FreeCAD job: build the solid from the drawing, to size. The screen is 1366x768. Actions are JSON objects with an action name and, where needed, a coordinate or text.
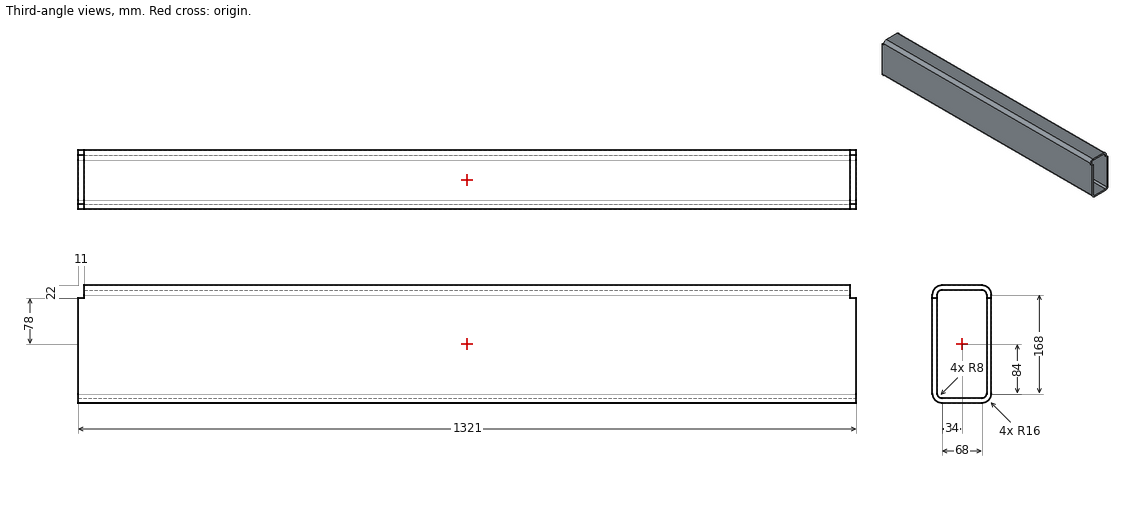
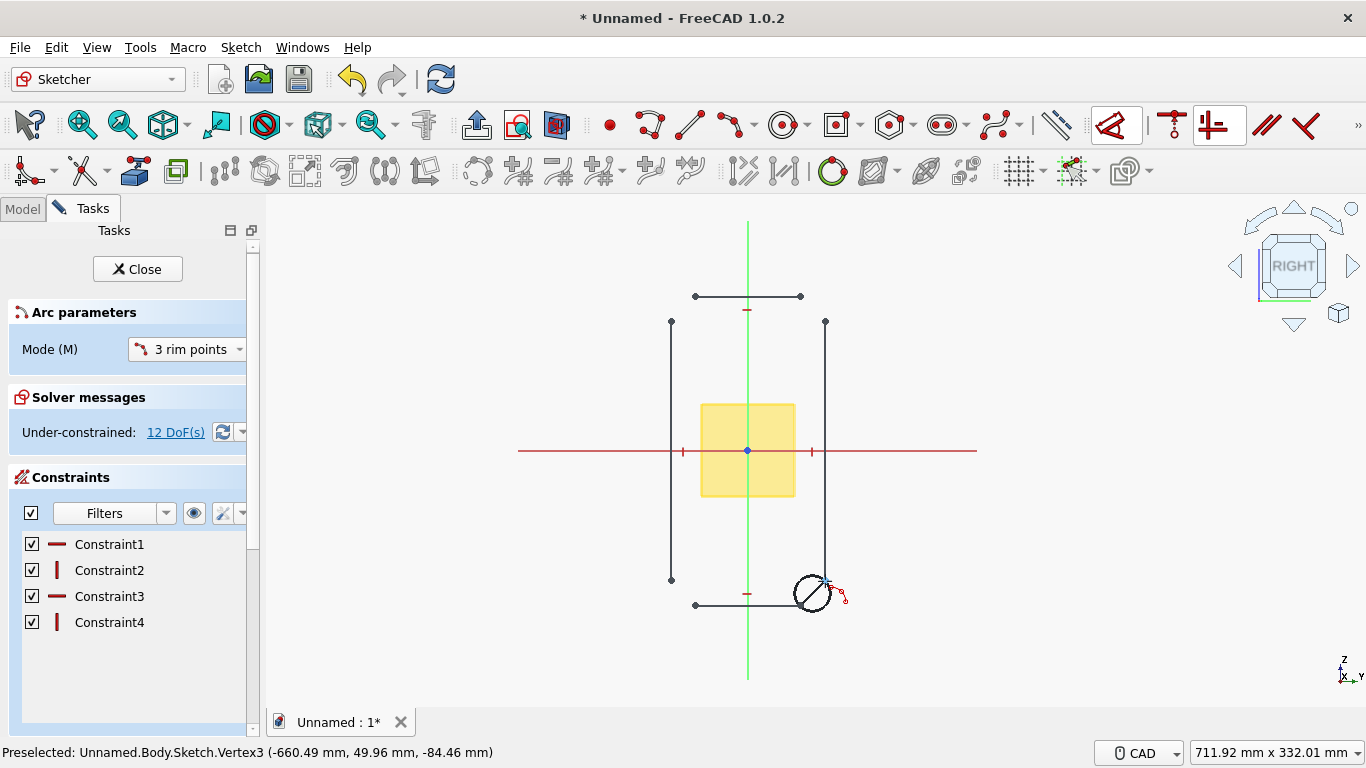
{"action": "scroll", "coordinate": [818, 598], "scroll_direction": "up", "scroll_amount": 4}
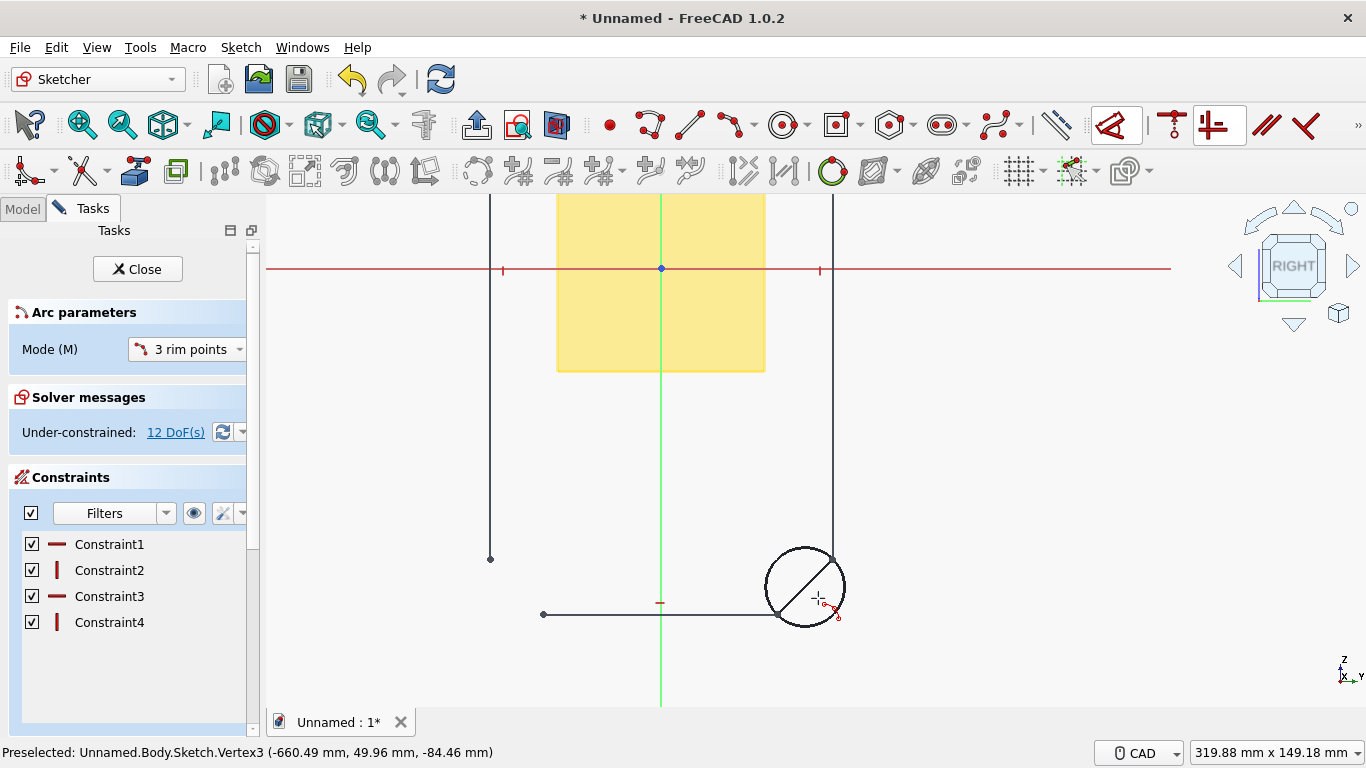
{"action": "left_click", "coordinate": [817, 597]}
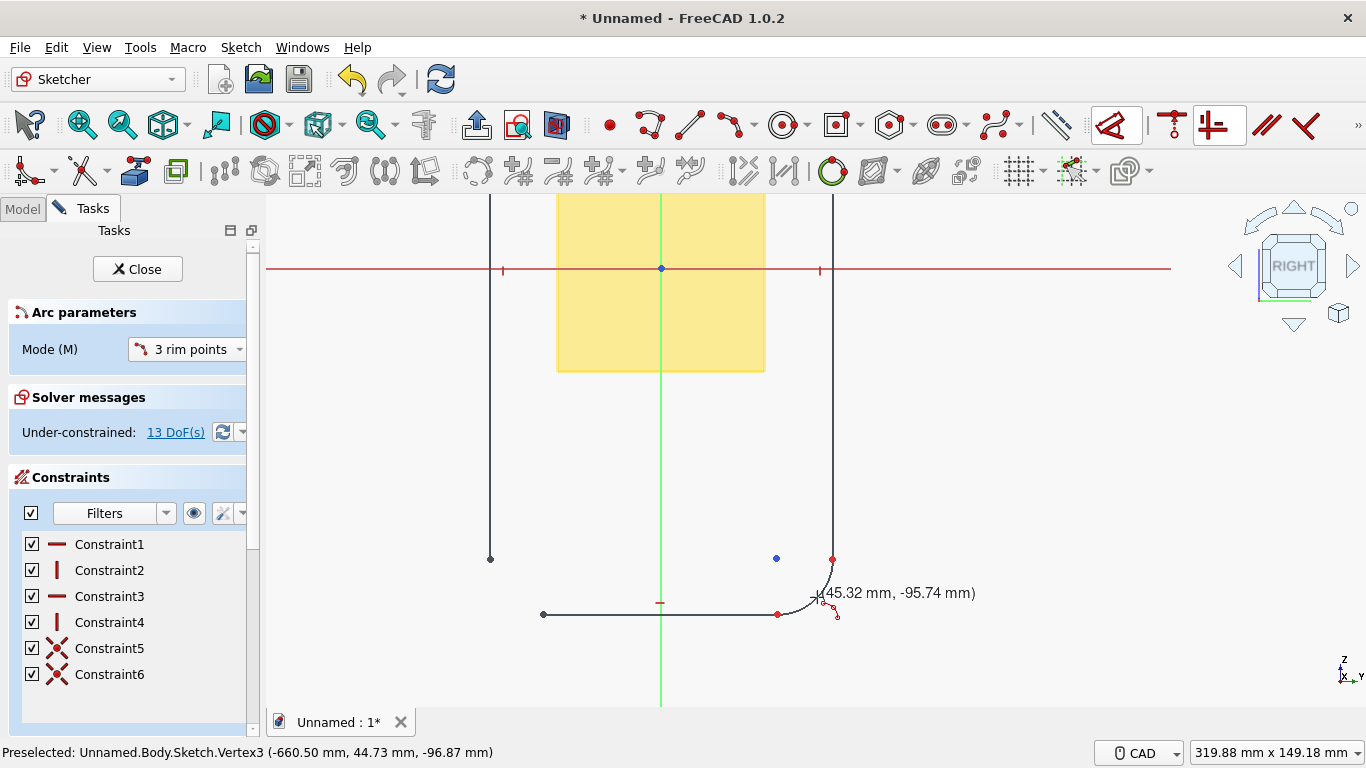
{"action": "scroll", "coordinate": [818, 599], "scroll_direction": "down", "scroll_amount": 4}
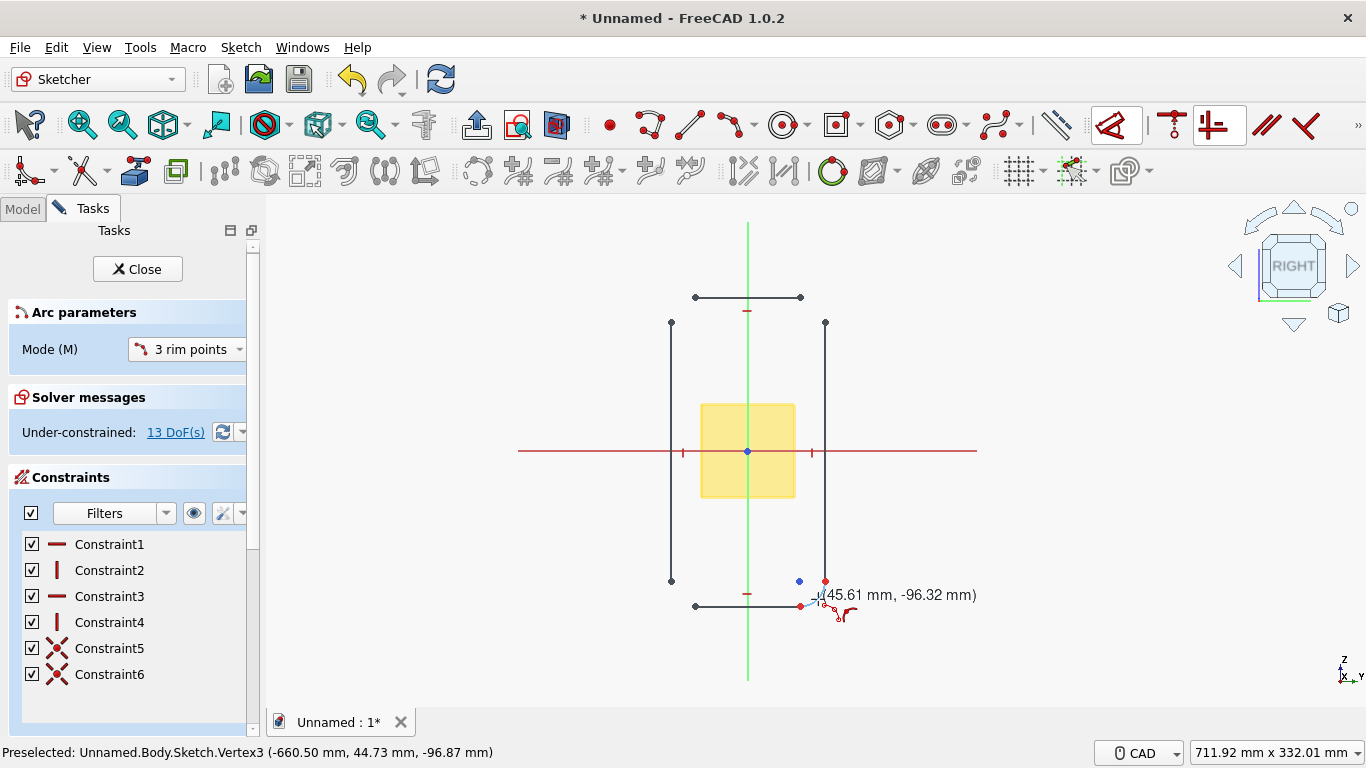
{"action": "left_click", "coordinate": [825, 323]}
{"action": "left_click", "coordinate": [800, 298]}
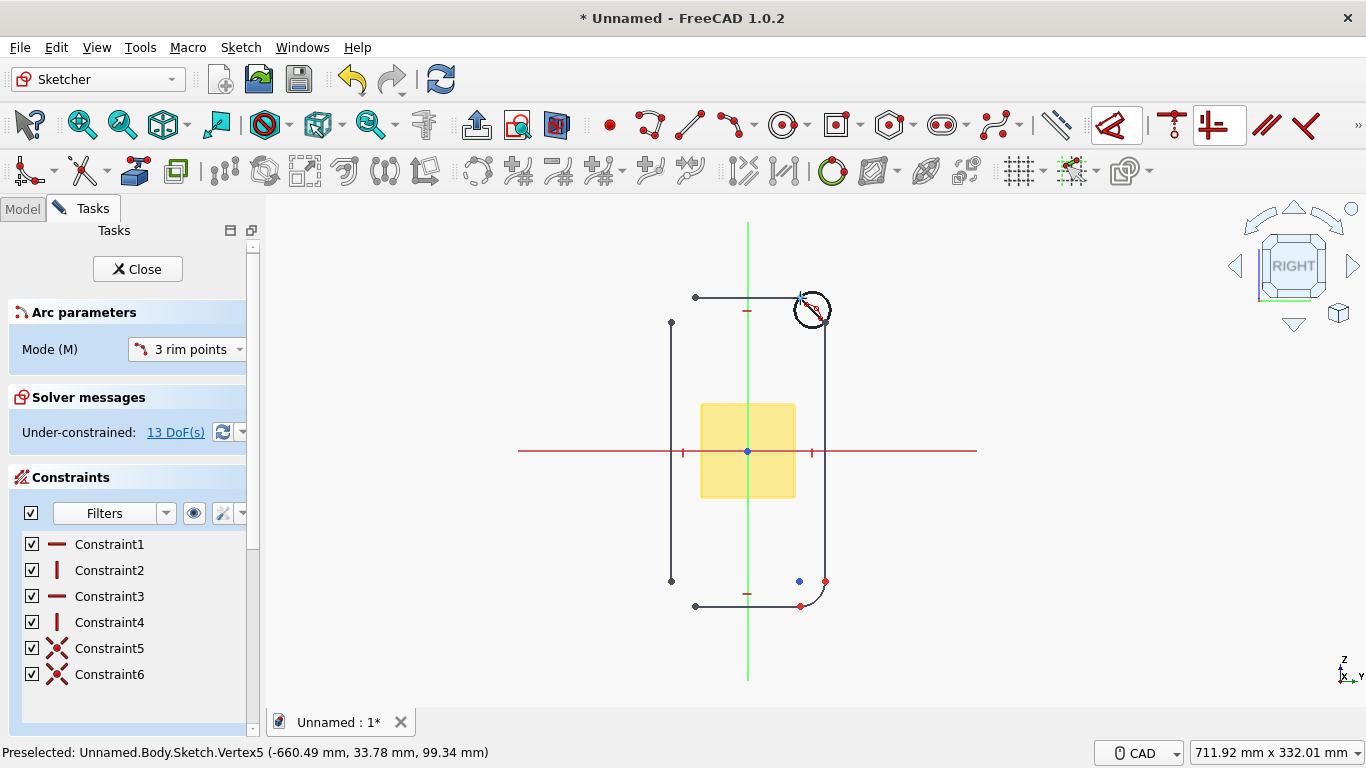
{"action": "scroll", "coordinate": [818, 304], "scroll_direction": "up", "scroll_amount": 4}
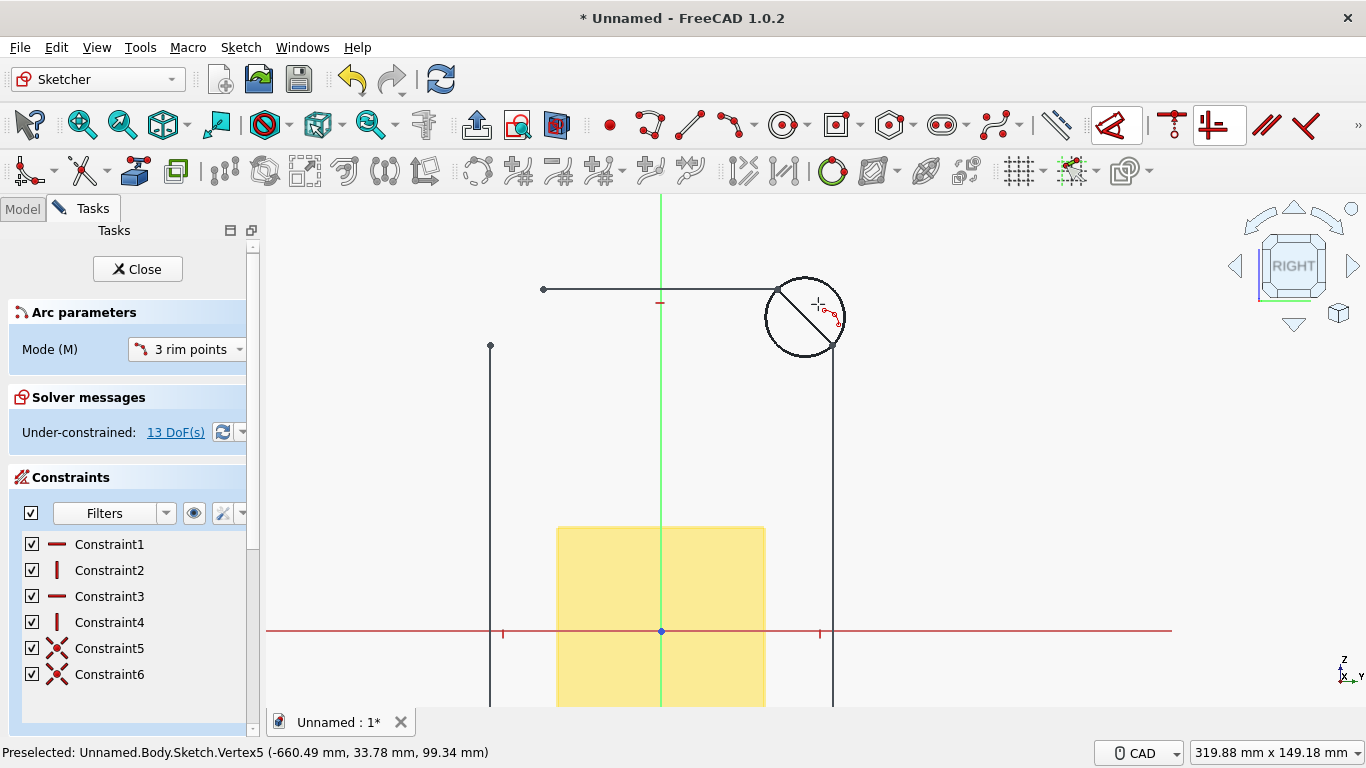
{"action": "left_click", "coordinate": [817, 303]}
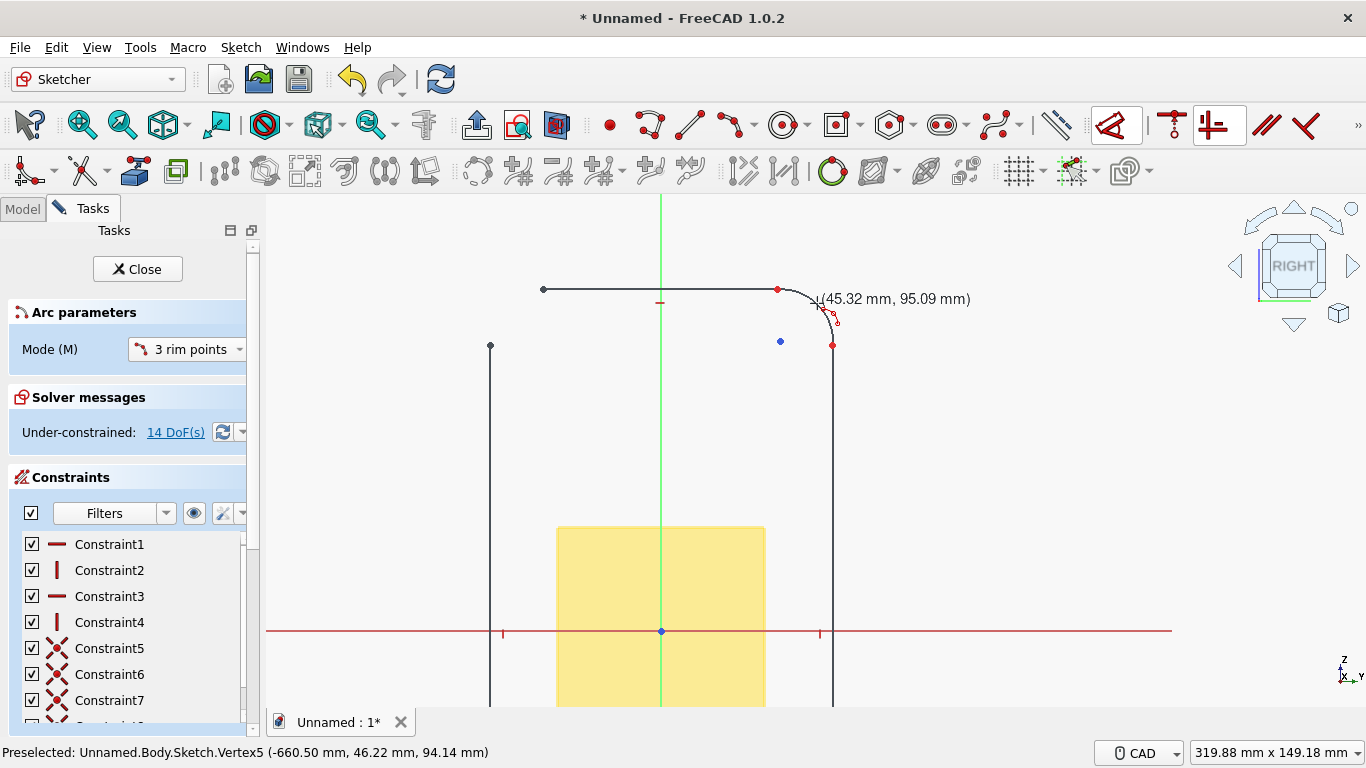
{"action": "left_click", "coordinate": [544, 289]}
{"action": "left_click", "coordinate": [490, 345]}
{"action": "left_click", "coordinate": [505, 303]}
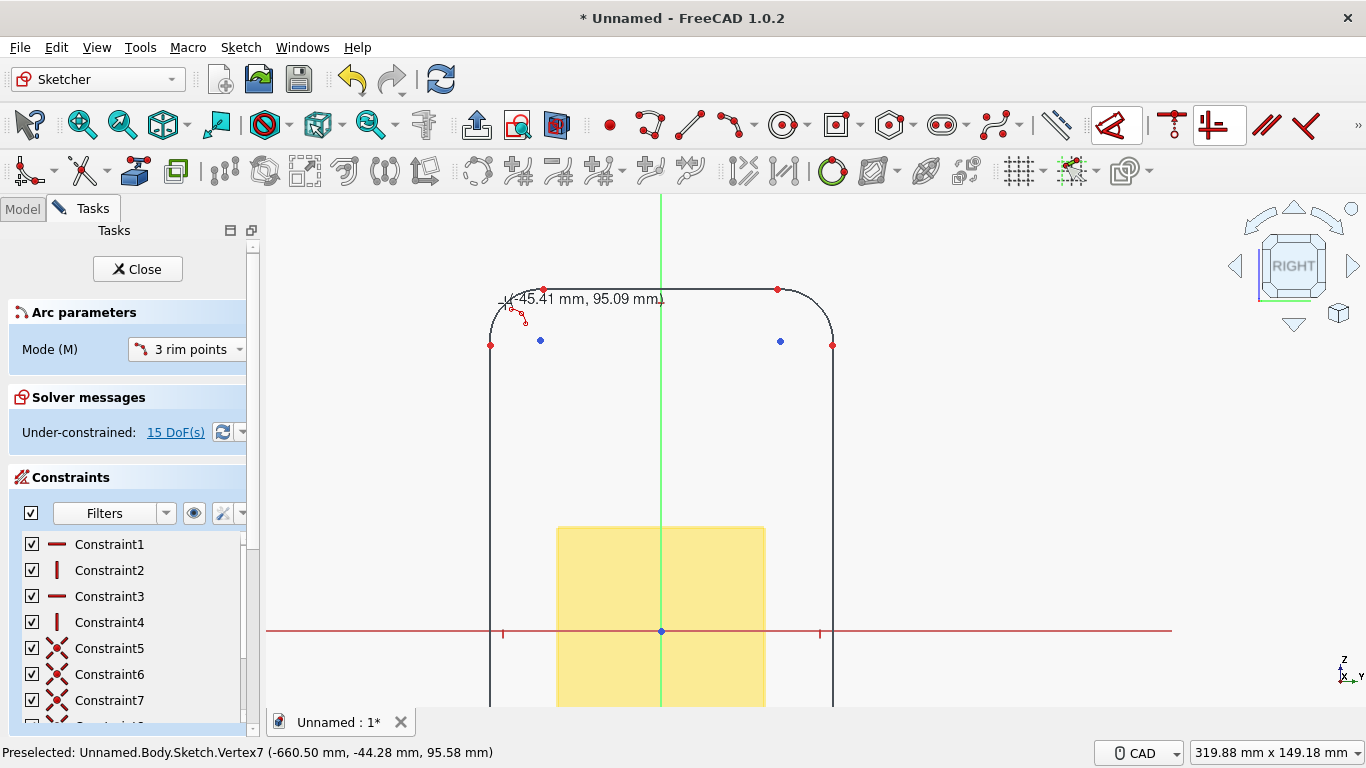
{"action": "scroll", "coordinate": [818, 303], "scroll_direction": "down", "scroll_amount": 4}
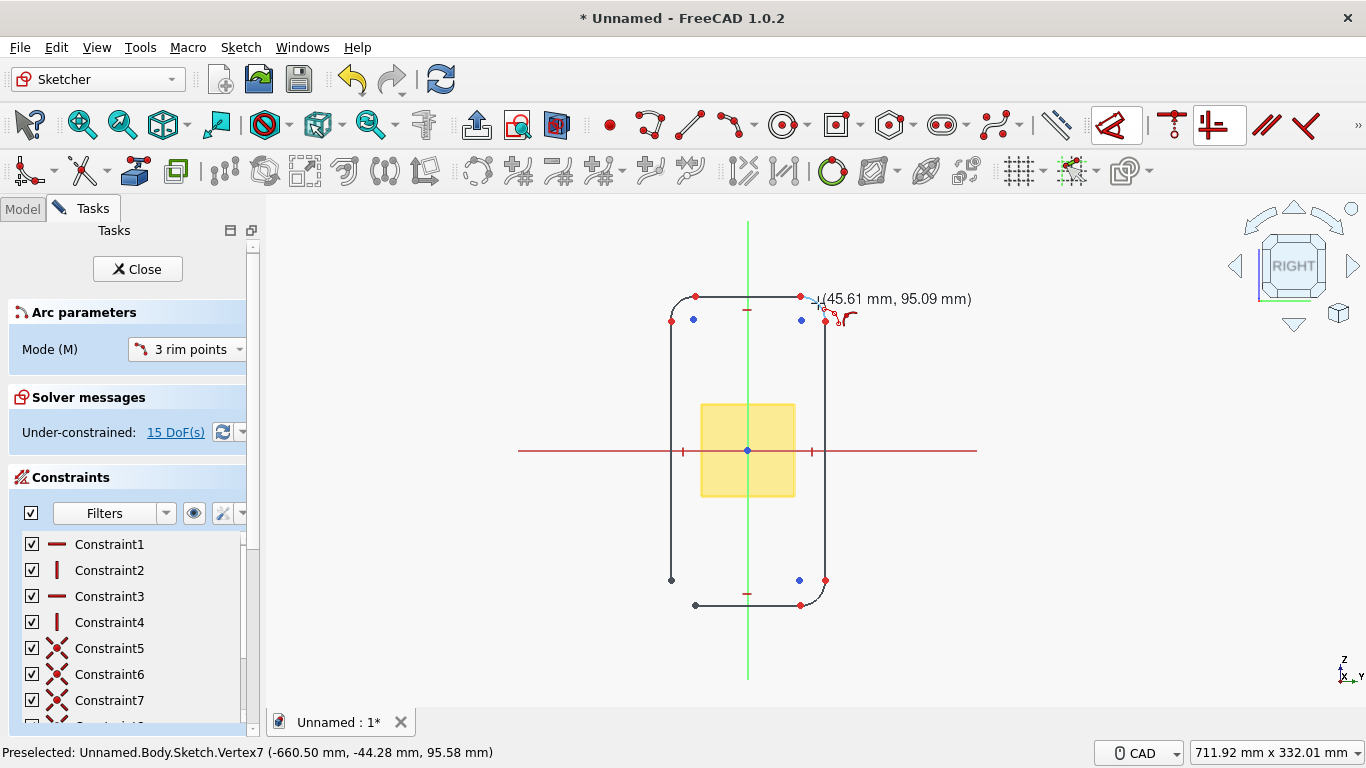
{"action": "left_click", "coordinate": [671, 581]}
{"action": "left_click", "coordinate": [695, 606]}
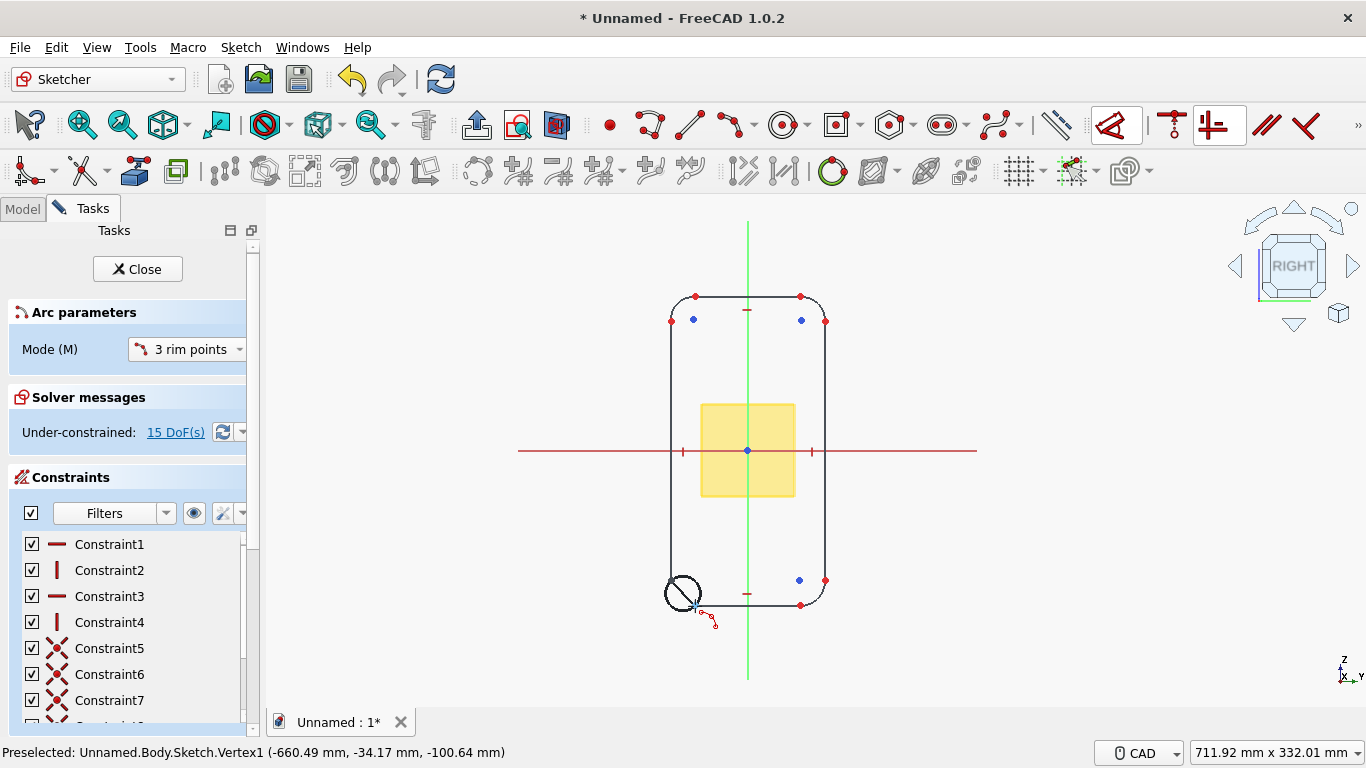
{"action": "scroll", "coordinate": [678, 598], "scroll_direction": "up", "scroll_amount": 4}